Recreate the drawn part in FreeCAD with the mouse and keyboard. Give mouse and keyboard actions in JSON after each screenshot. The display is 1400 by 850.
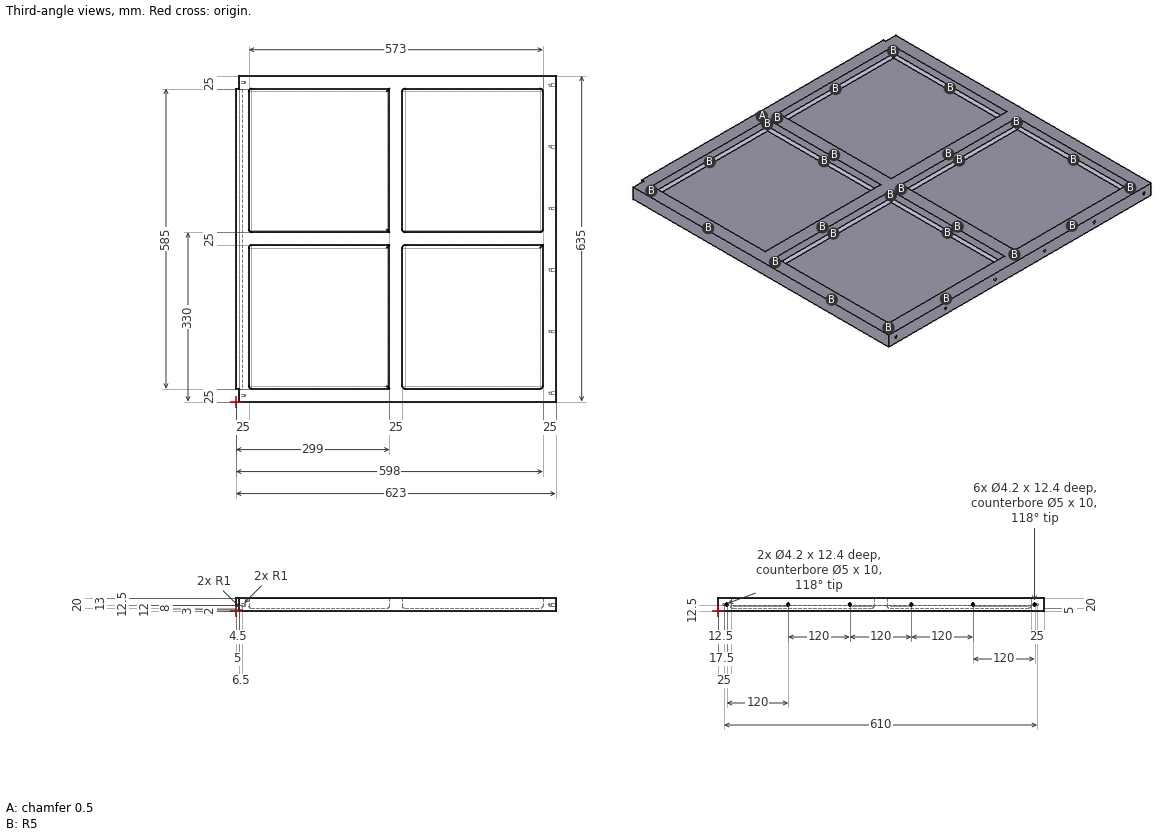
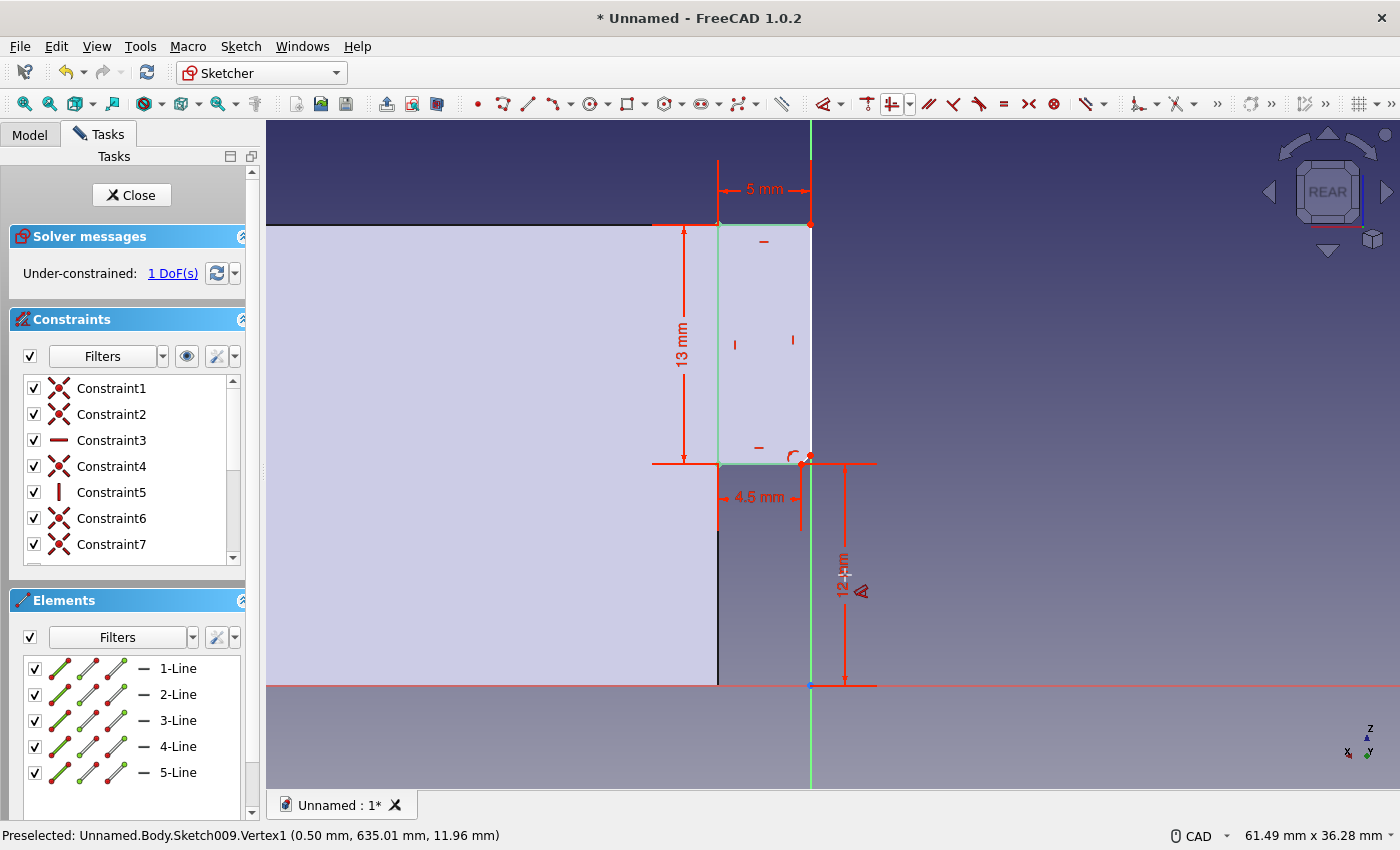
{"action": "left_click", "coordinate": [811, 386]}
{"action": "left_click", "coordinate": [845, 340]}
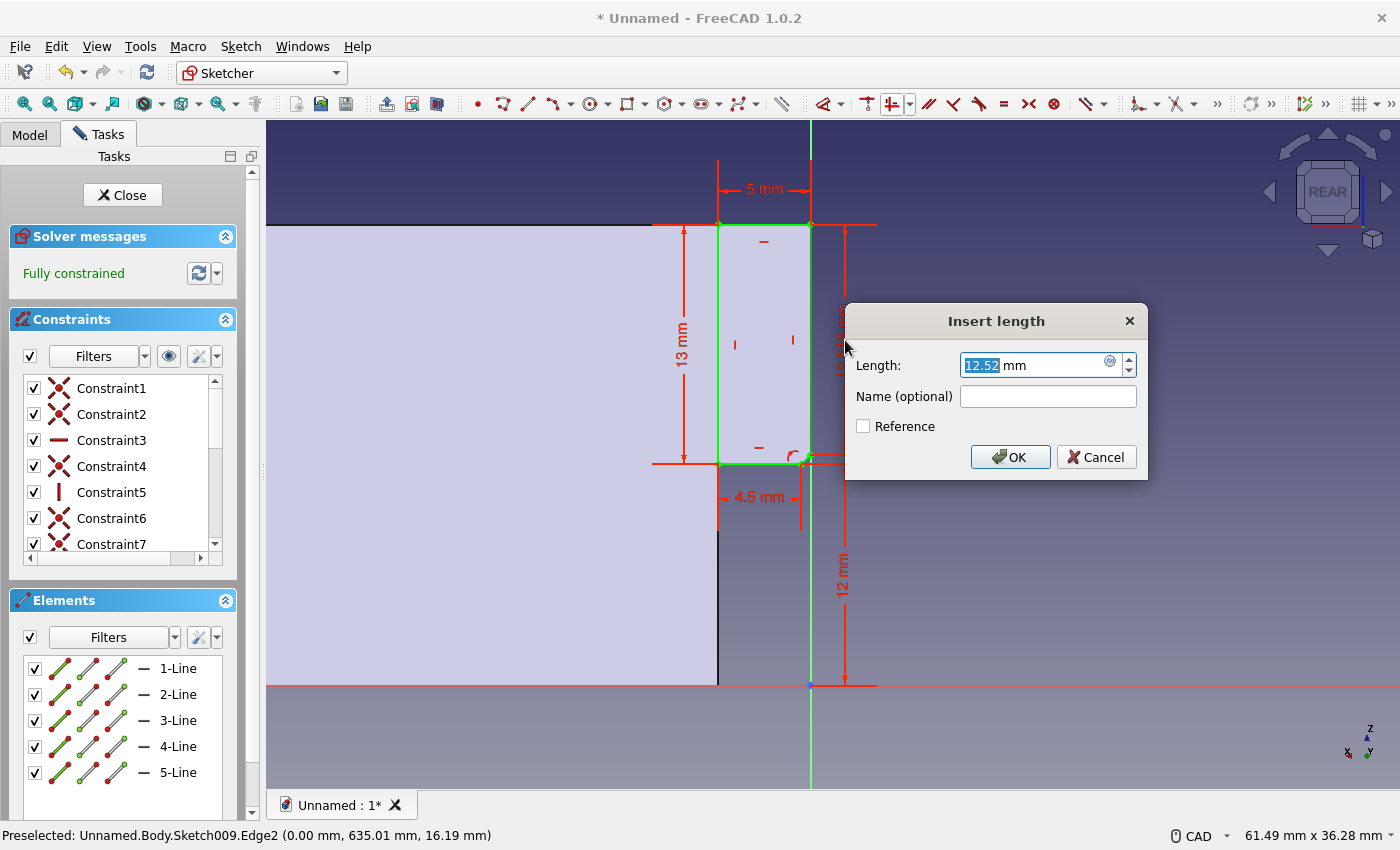
{"action": "type", "text": "12.5"}
{"action": "key", "text": "Return"}
{"action": "key", "text": "Escape"}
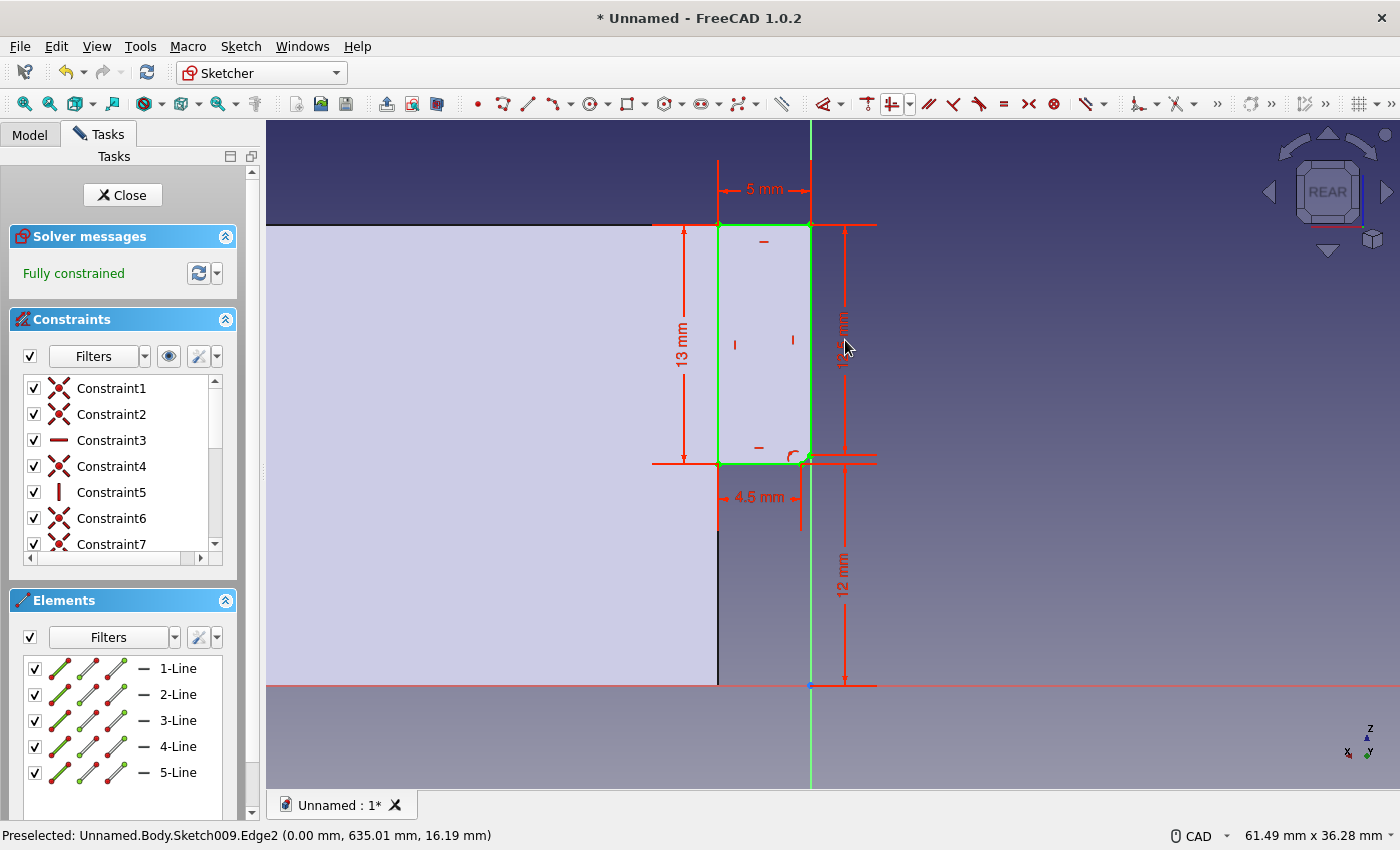
{"action": "left_click", "coordinate": [123, 195]}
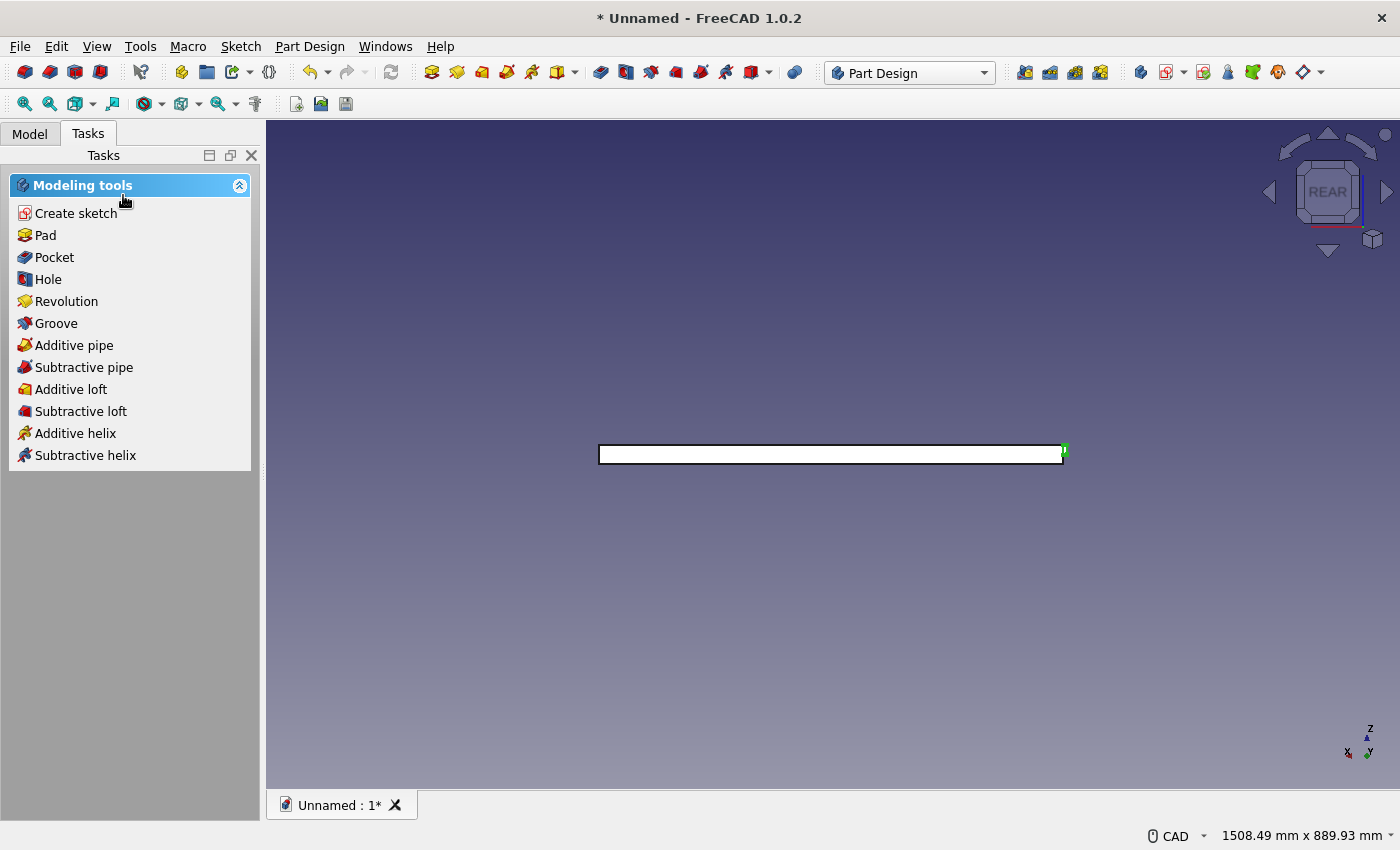
{"action": "left_click", "coordinate": [601, 72]}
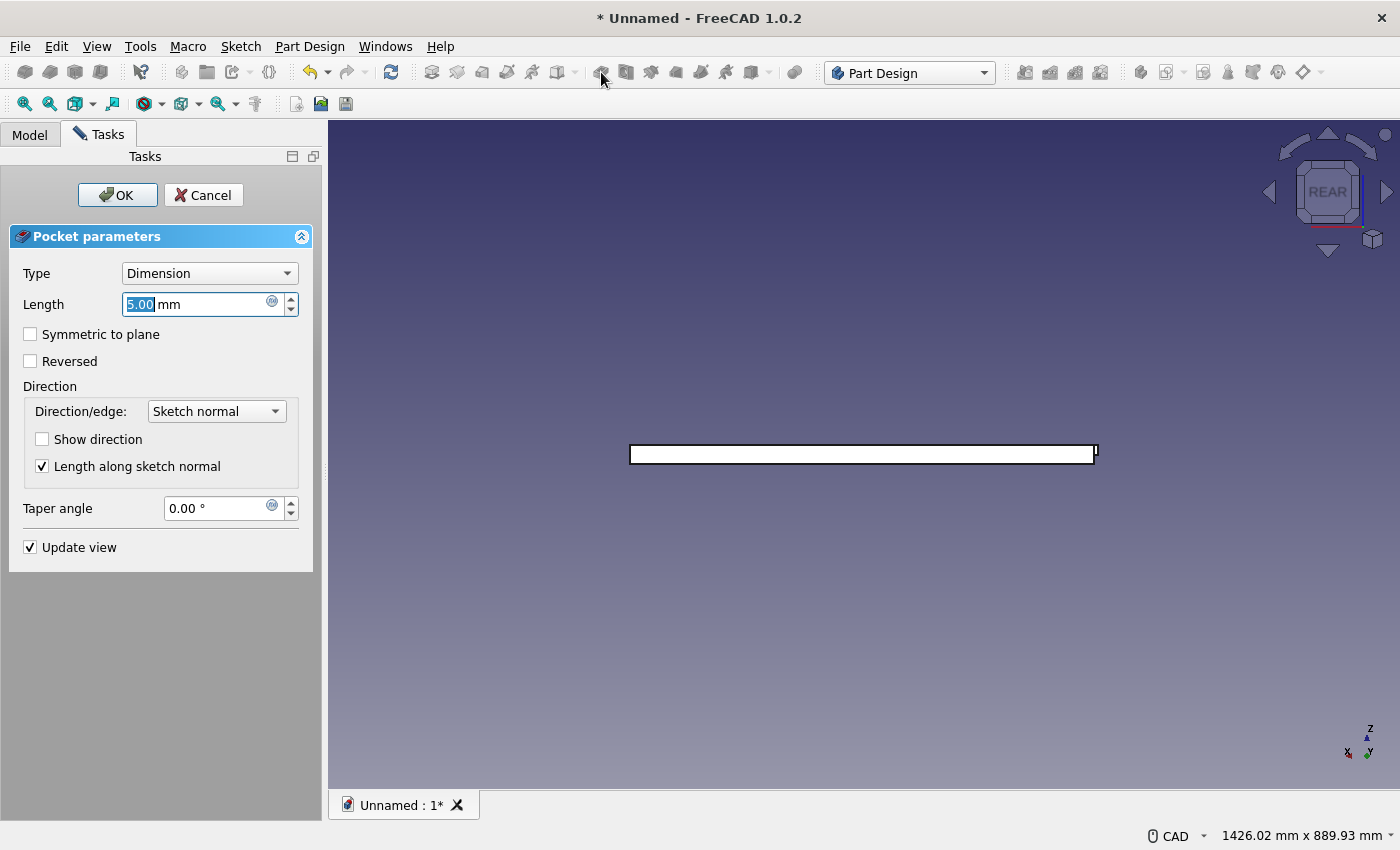
{"action": "type", "text": "25"}
{"action": "key", "text": "Tab"}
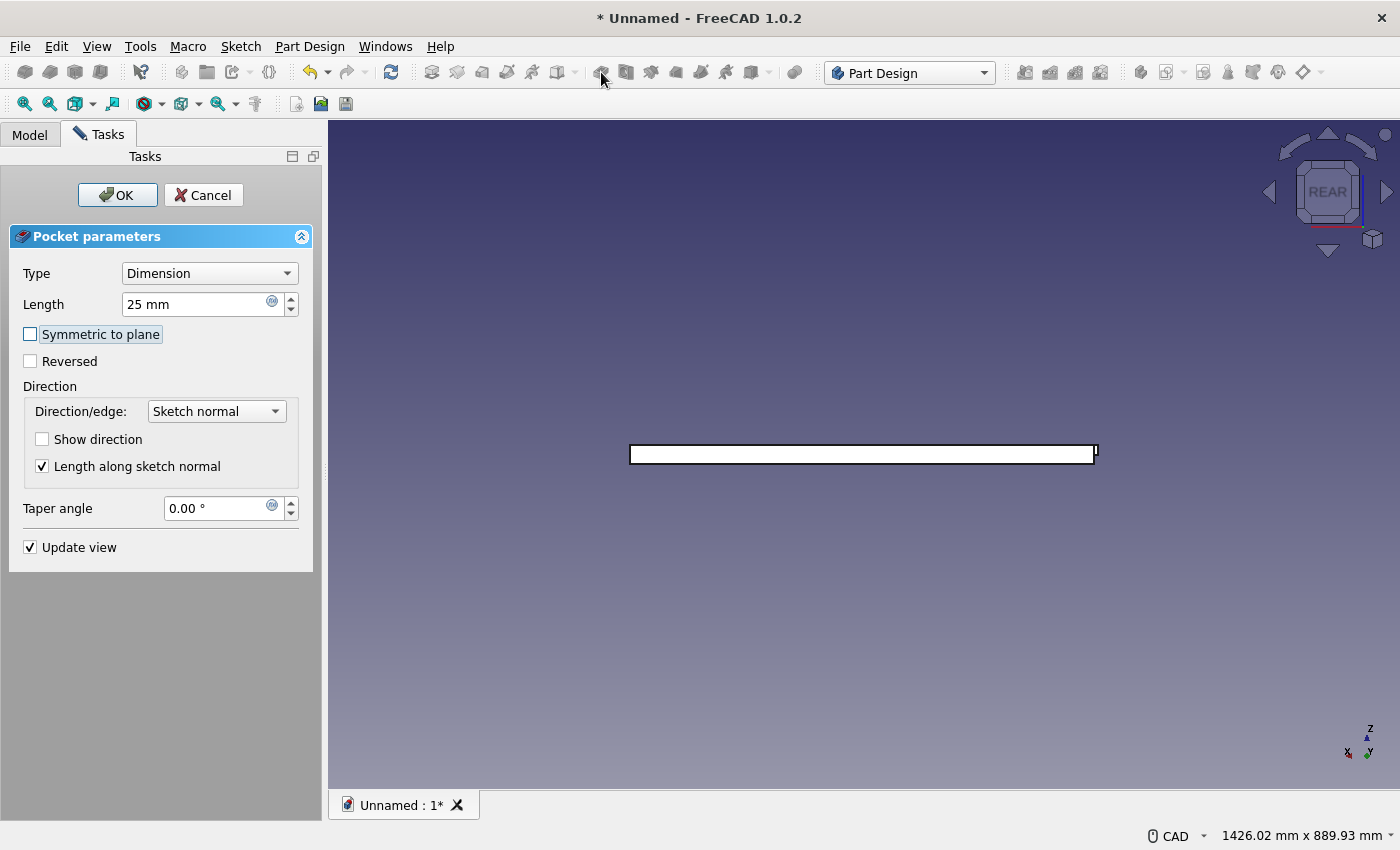
{"action": "left_click", "coordinate": [118, 195]}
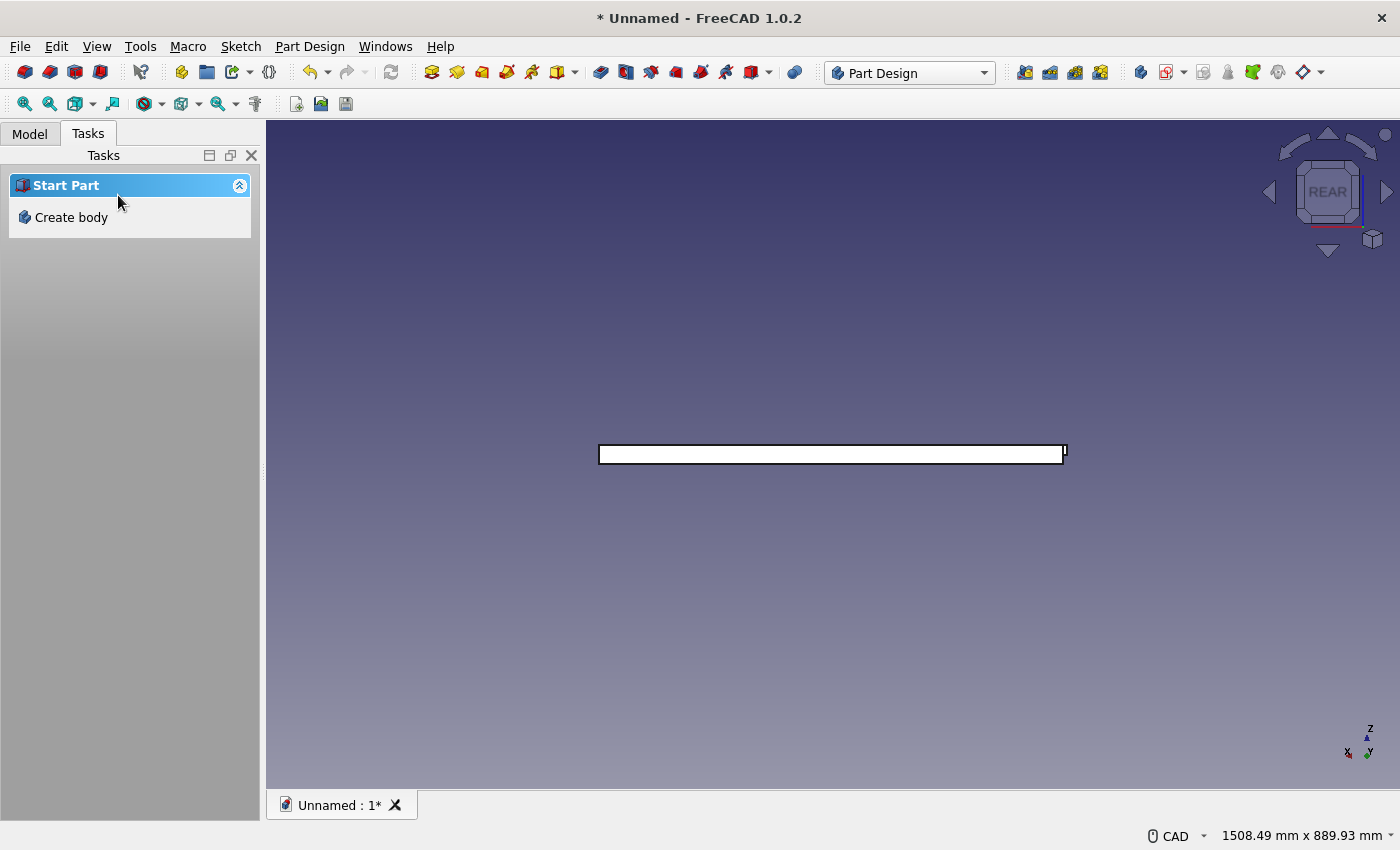
{"action": "key", "text": "v f"}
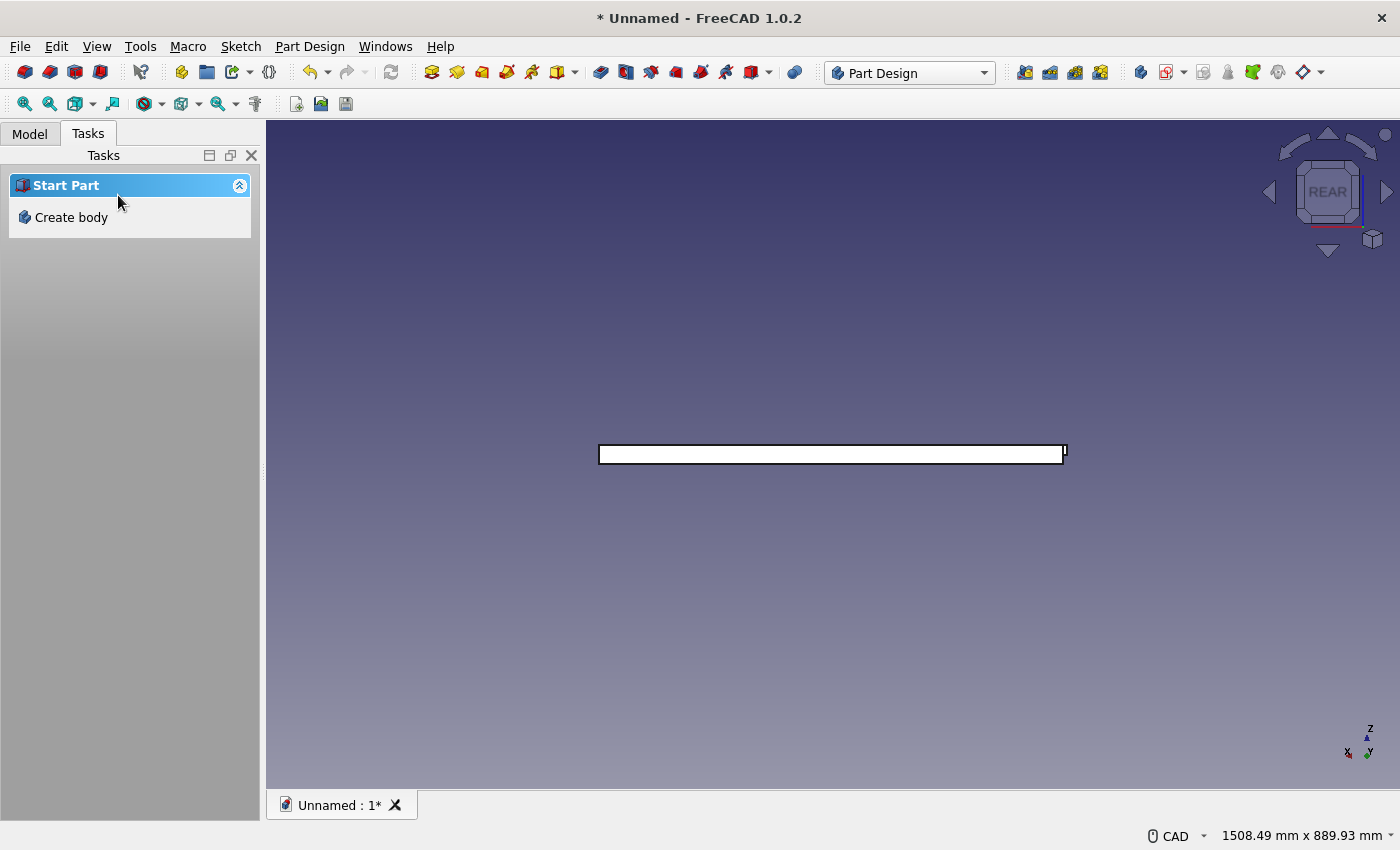
{"action": "left_click", "coordinate": [30, 134]}